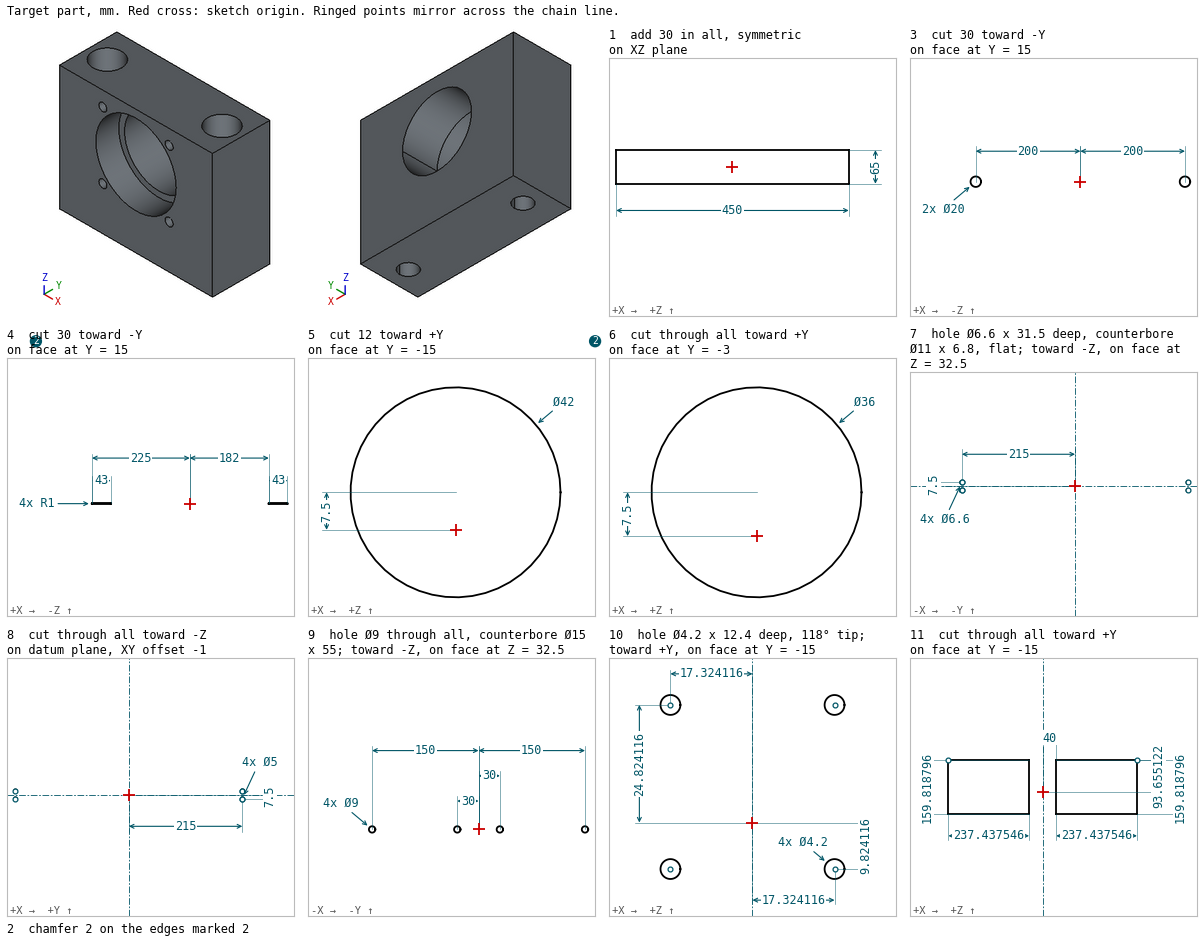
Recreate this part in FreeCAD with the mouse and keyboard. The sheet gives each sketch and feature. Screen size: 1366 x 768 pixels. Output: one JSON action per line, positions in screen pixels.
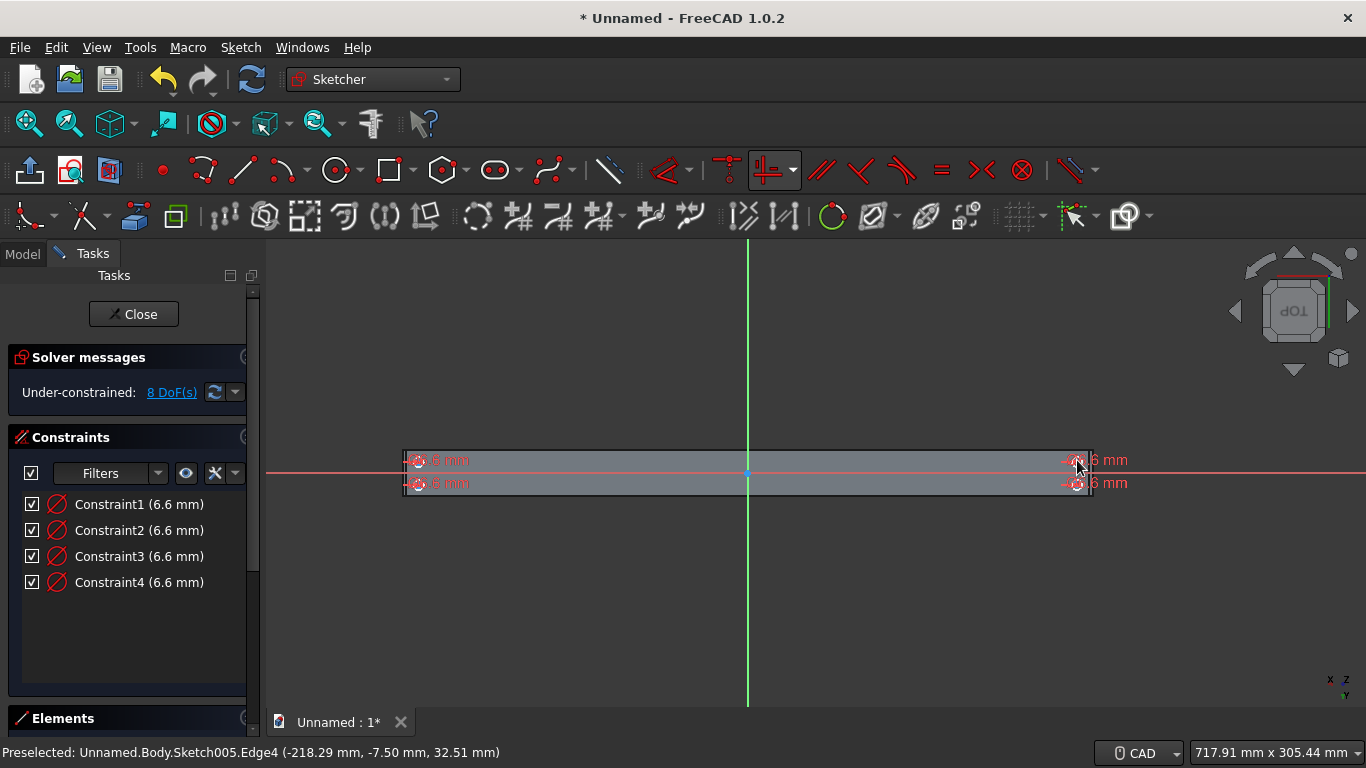
{"action": "left_click", "coordinate": [419, 462]}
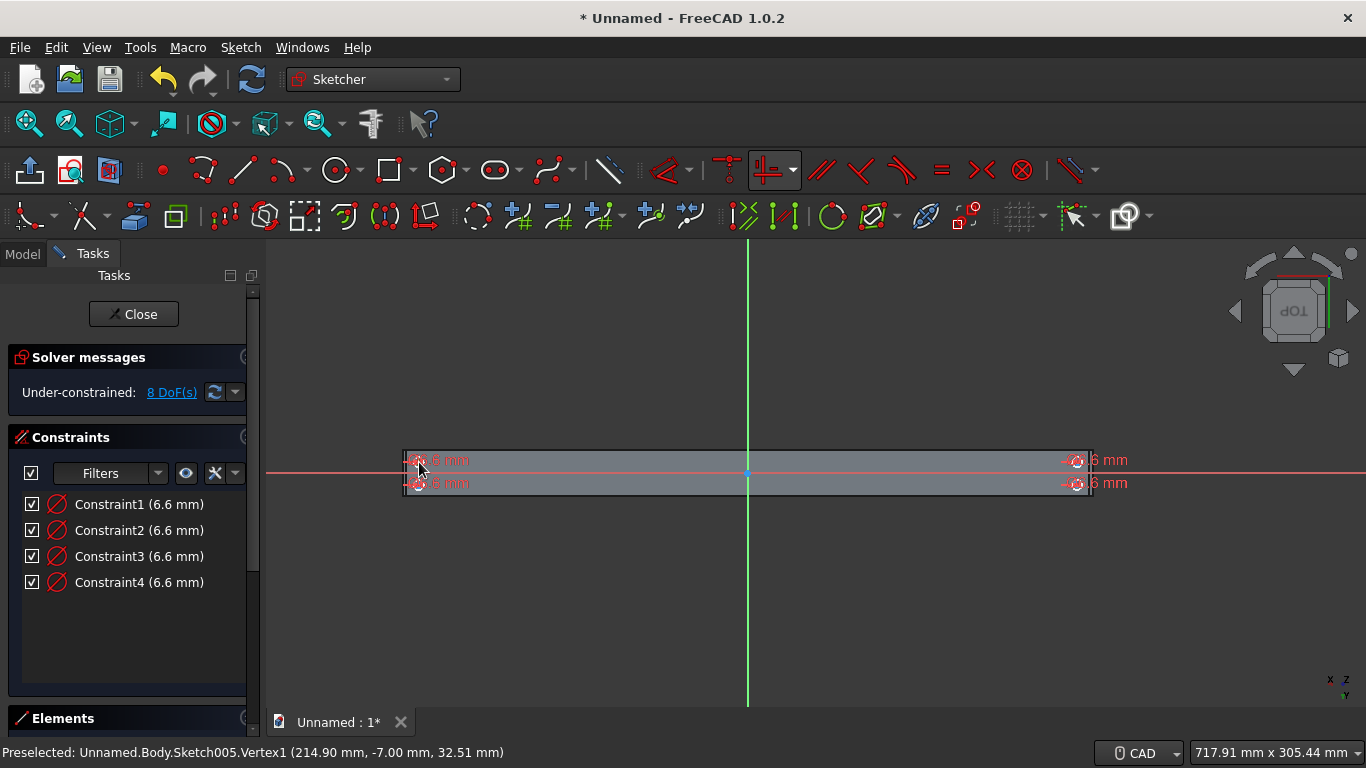
{"action": "left_click", "coordinate": [419, 485]}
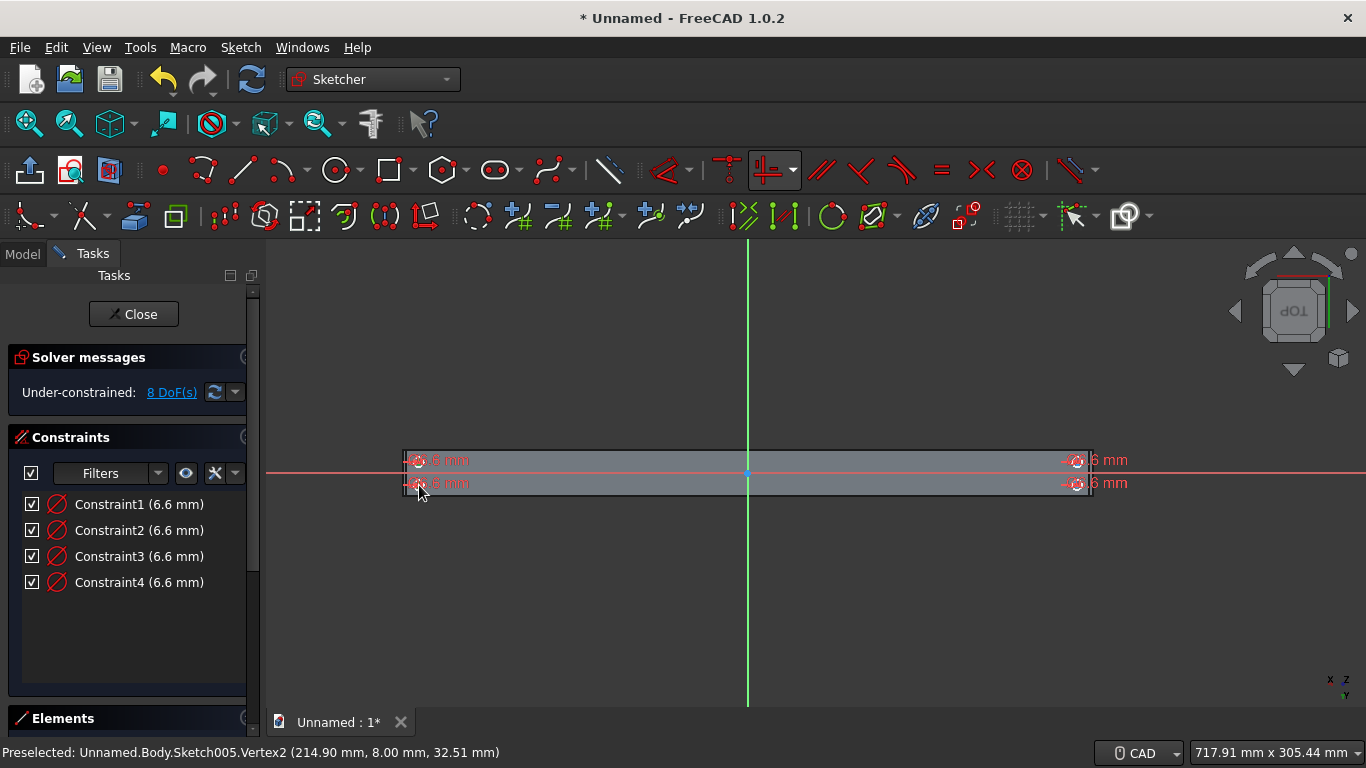
{"action": "left_click", "coordinate": [359, 473]}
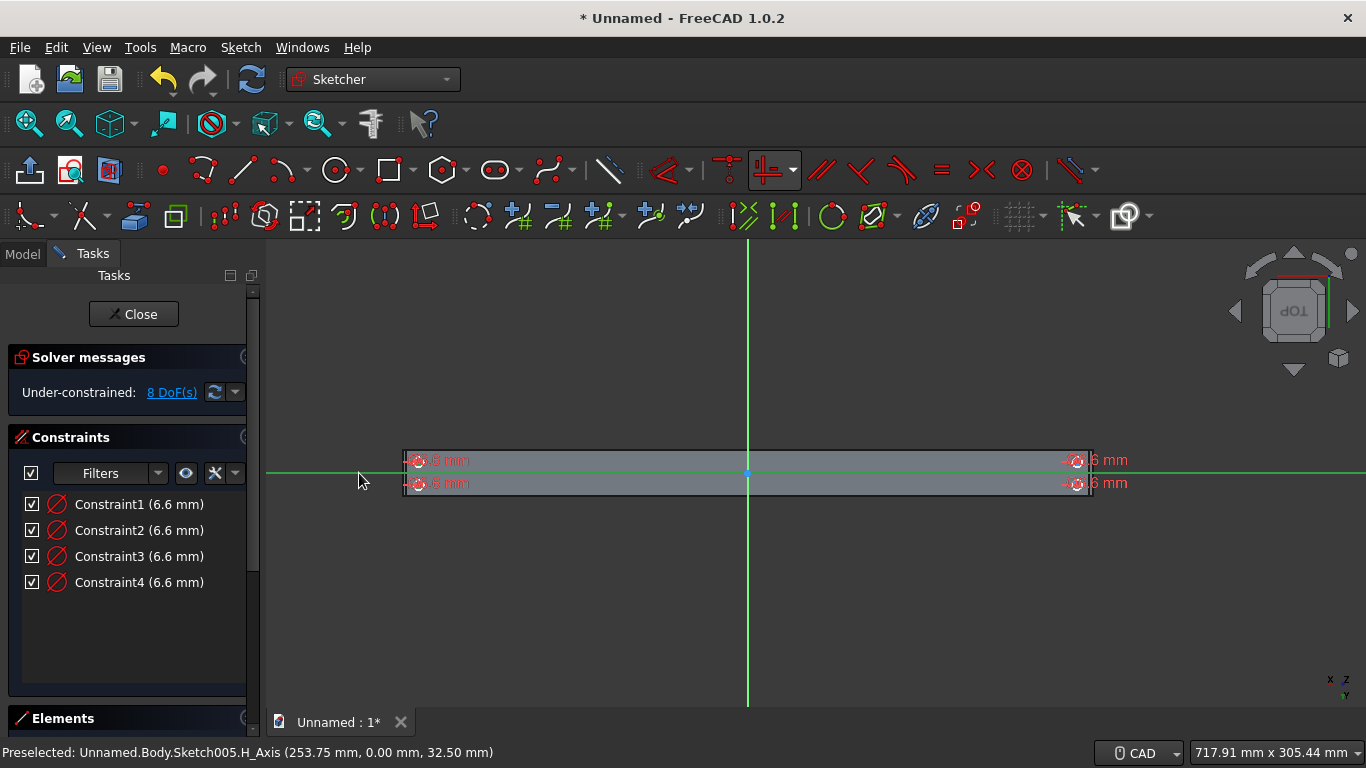
{"action": "left_click", "coordinate": [982, 170]}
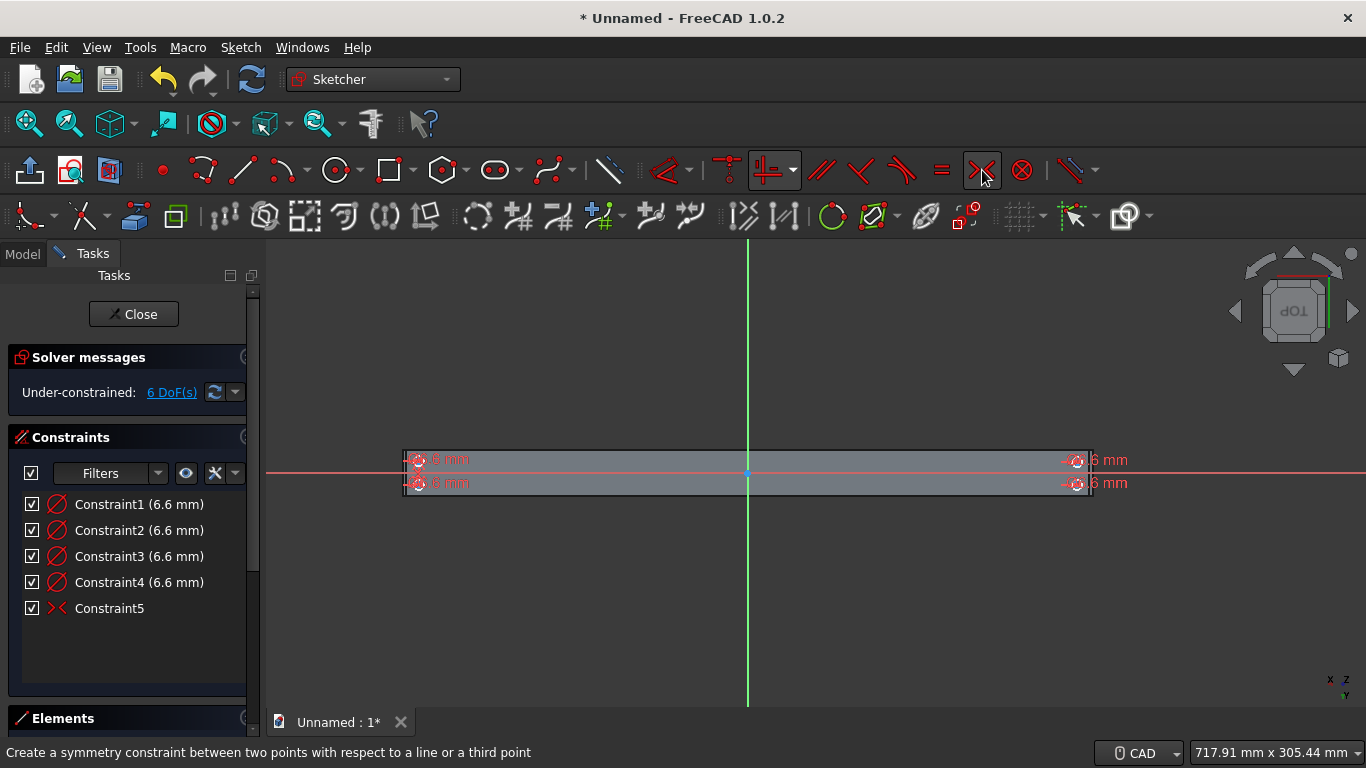
{"action": "left_click", "coordinate": [419, 485]}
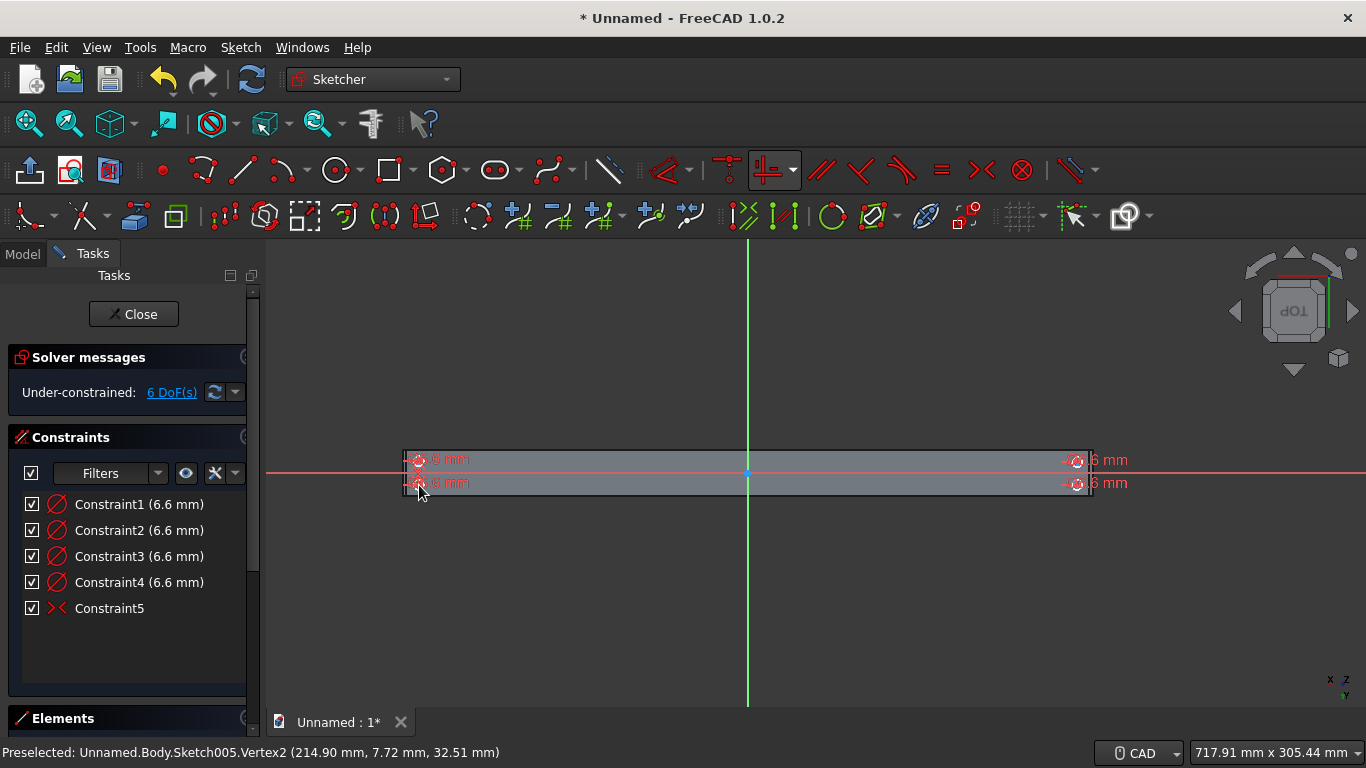
{"action": "left_click", "coordinate": [1077, 485]}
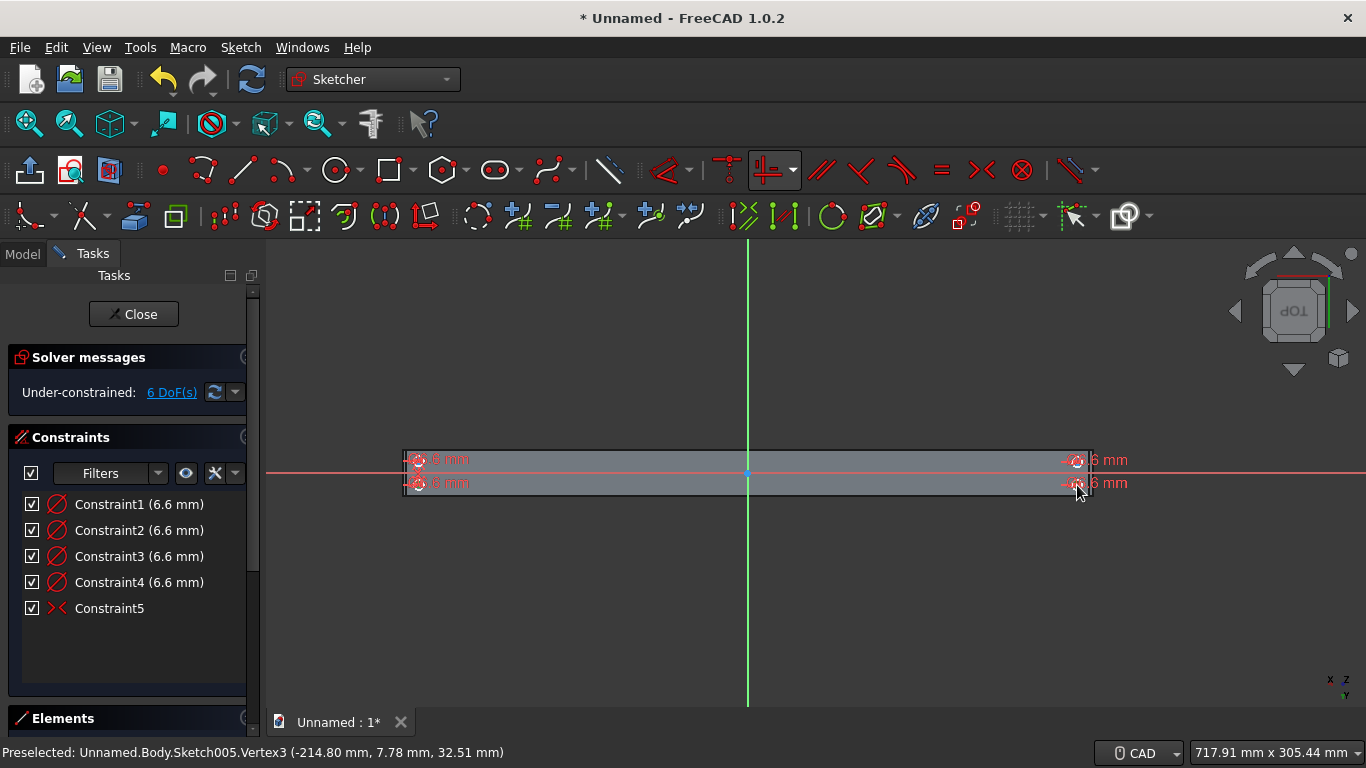
{"action": "left_click", "coordinate": [748, 650]}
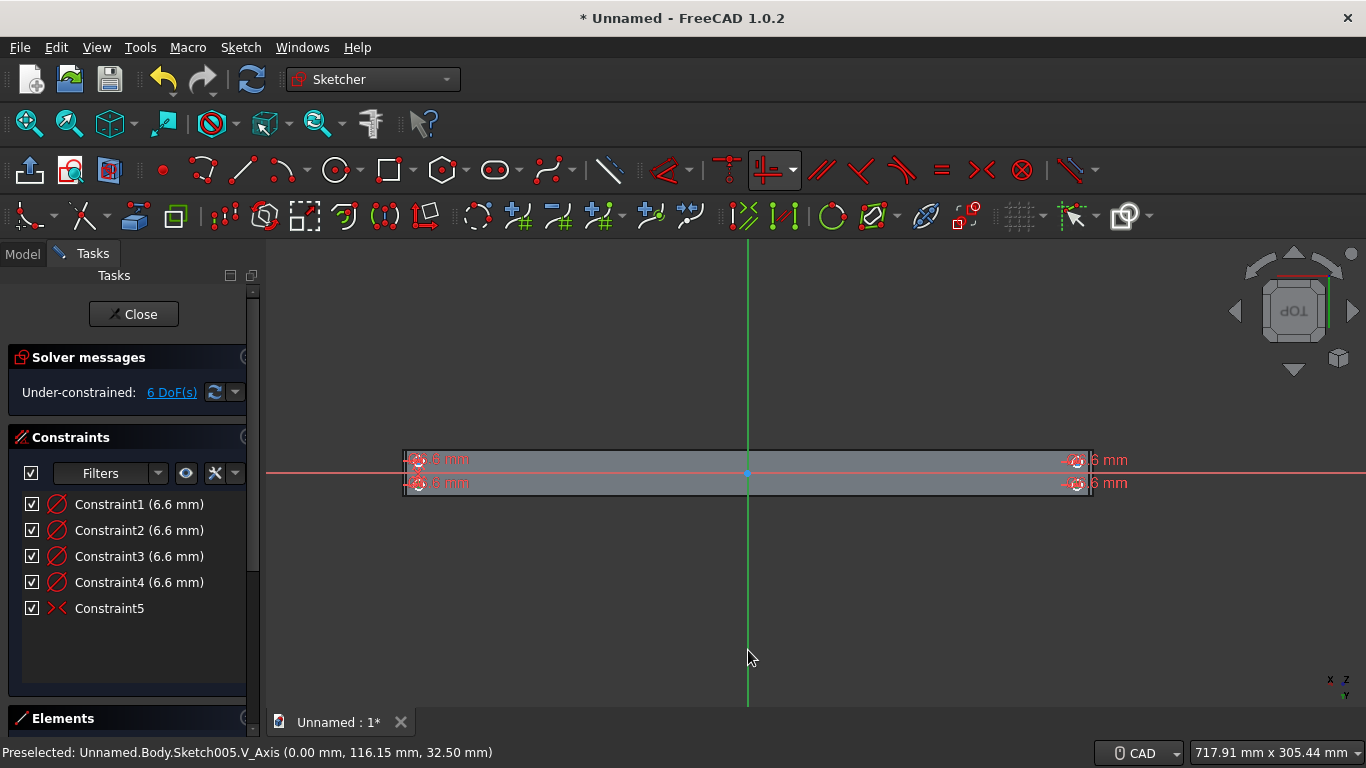
{"action": "key", "text": "s"}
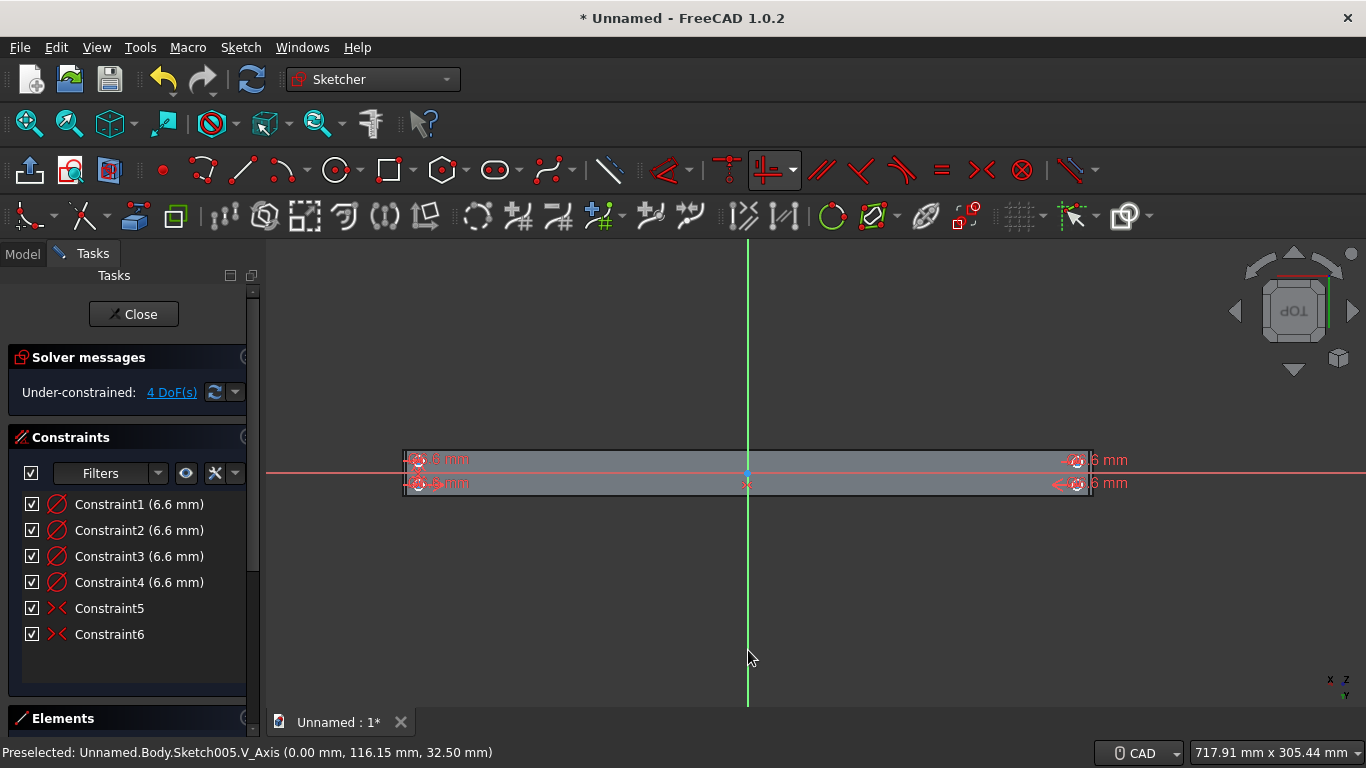
{"action": "left_click", "coordinate": [419, 461]}